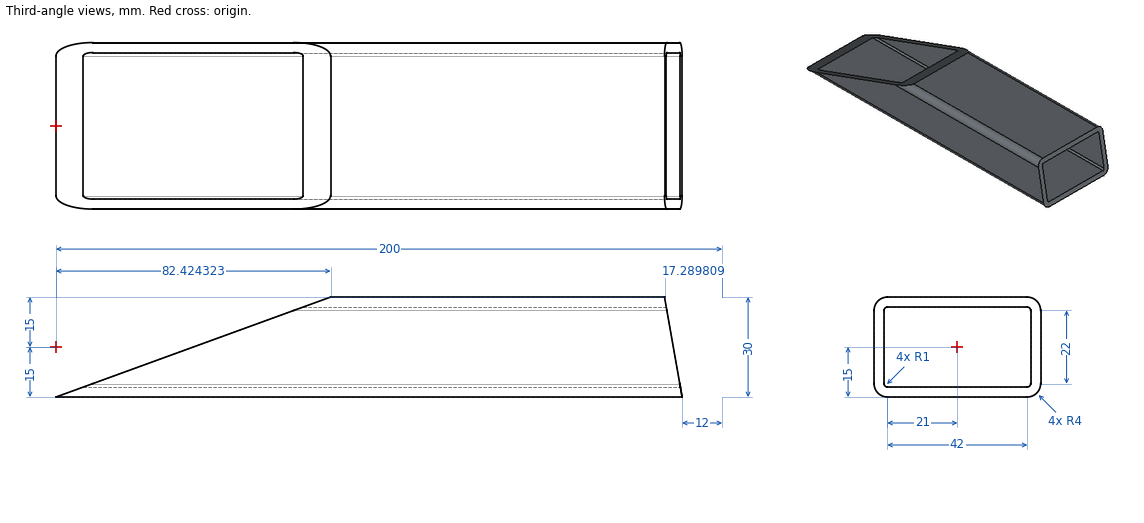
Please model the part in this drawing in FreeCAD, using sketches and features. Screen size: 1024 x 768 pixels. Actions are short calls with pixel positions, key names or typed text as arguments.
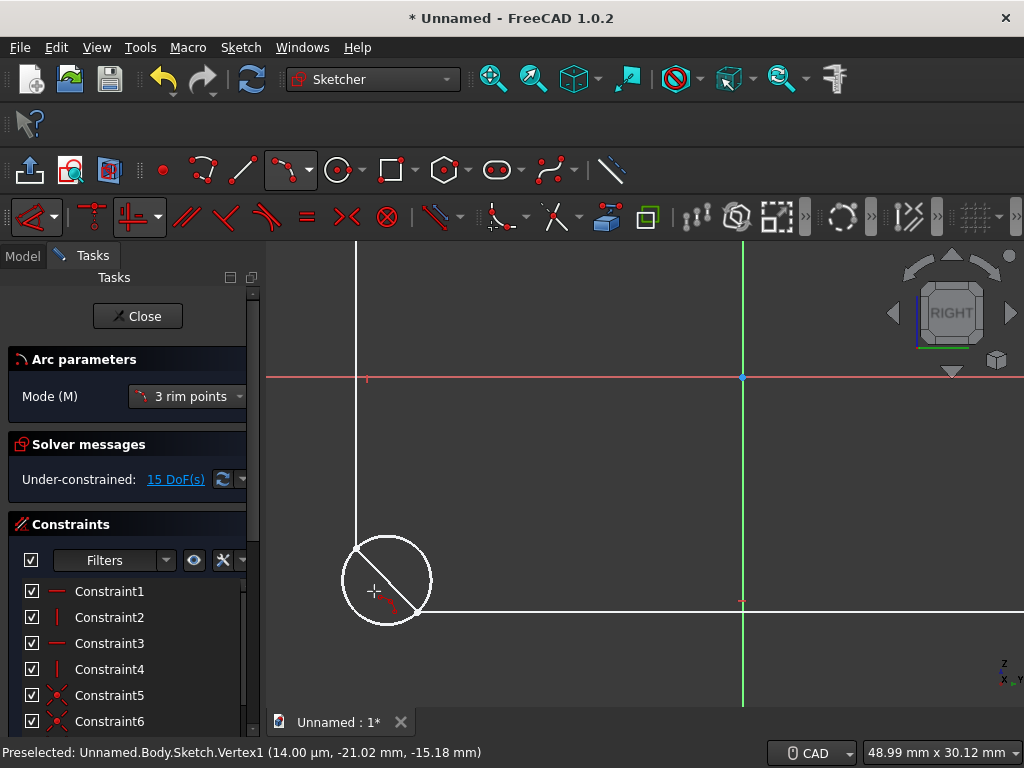
click(374, 591)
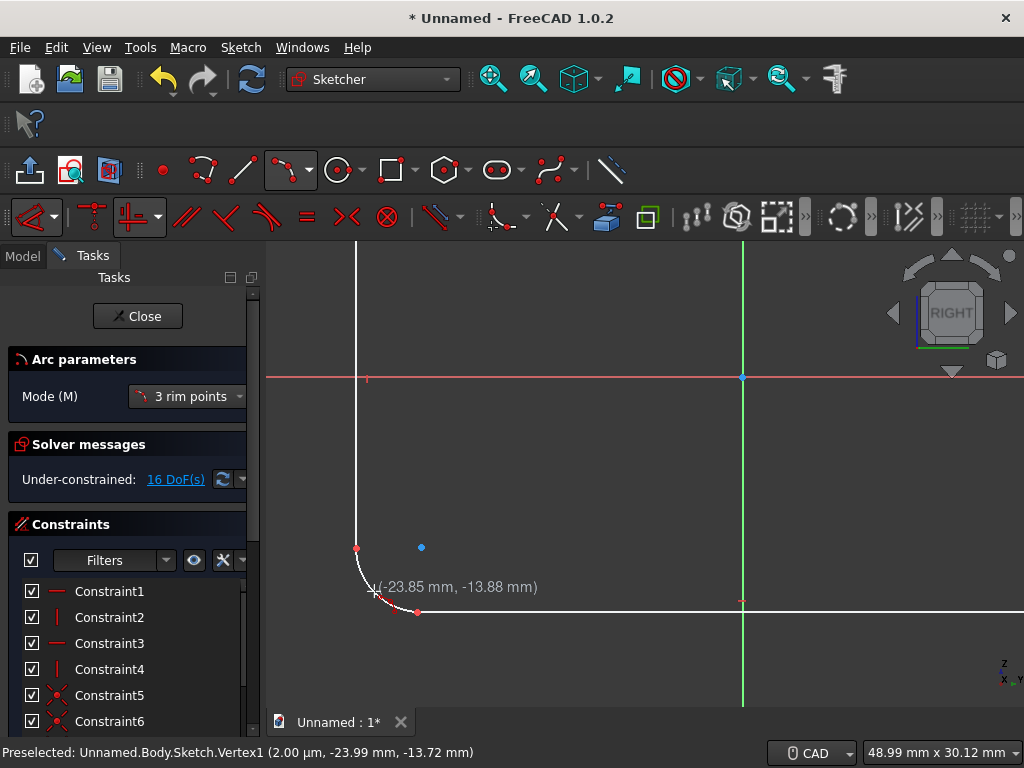
click(244, 170)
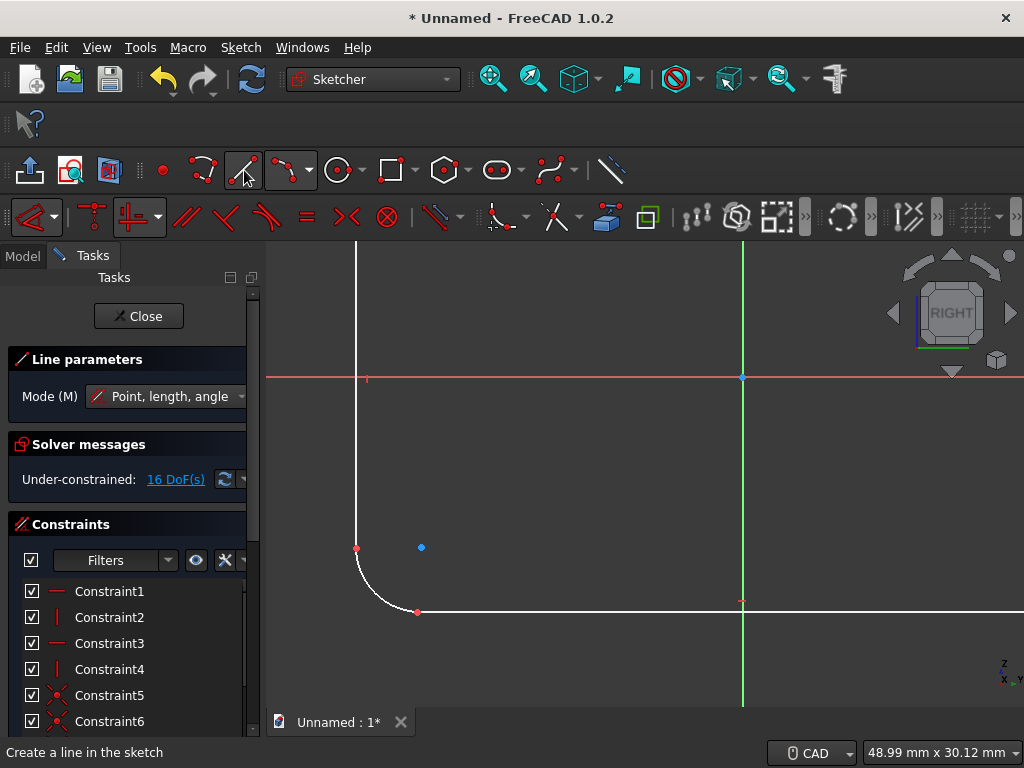
scroll(374, 592, down, 3)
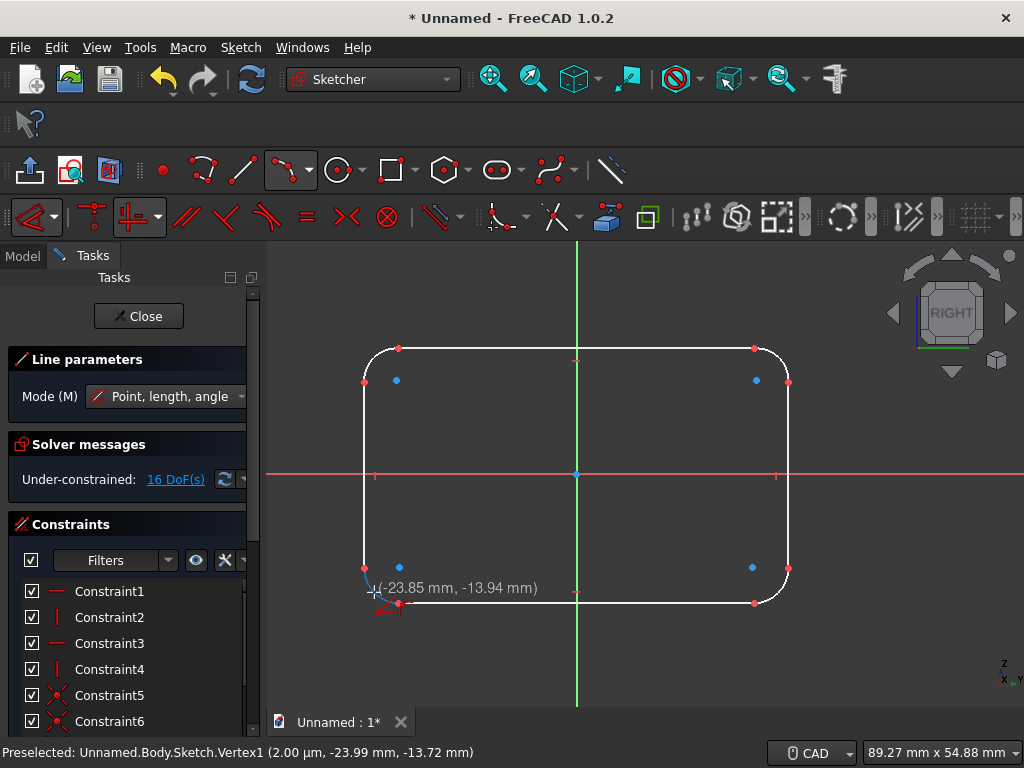
scroll(755, 576, up, 4)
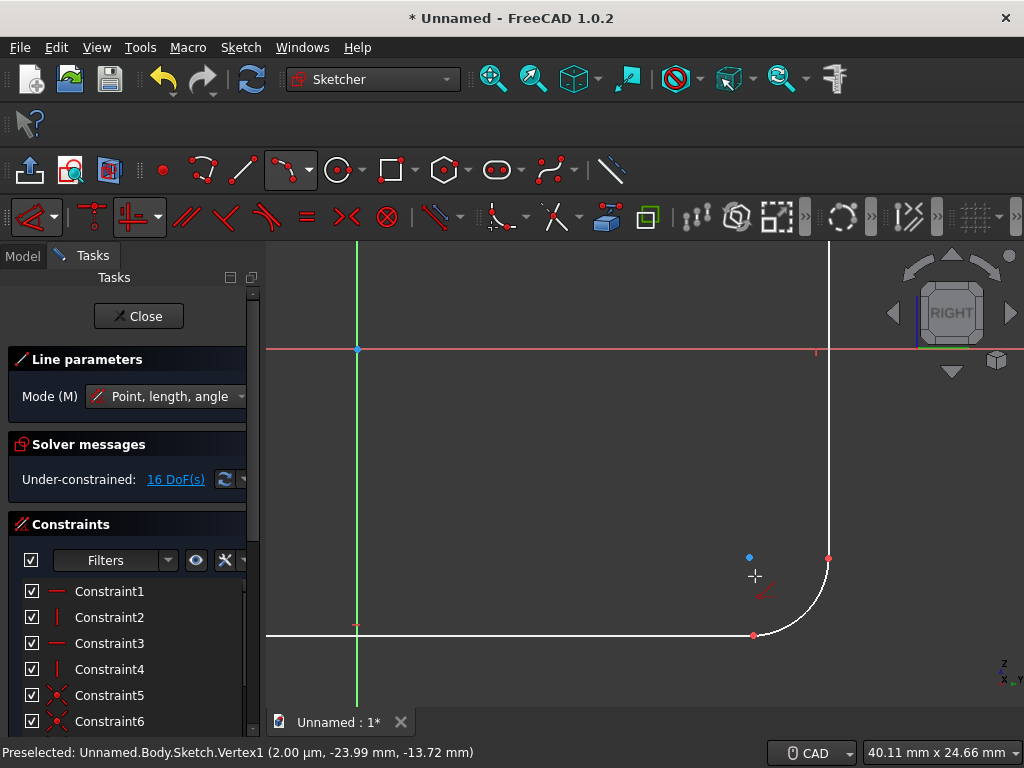
click(754, 576)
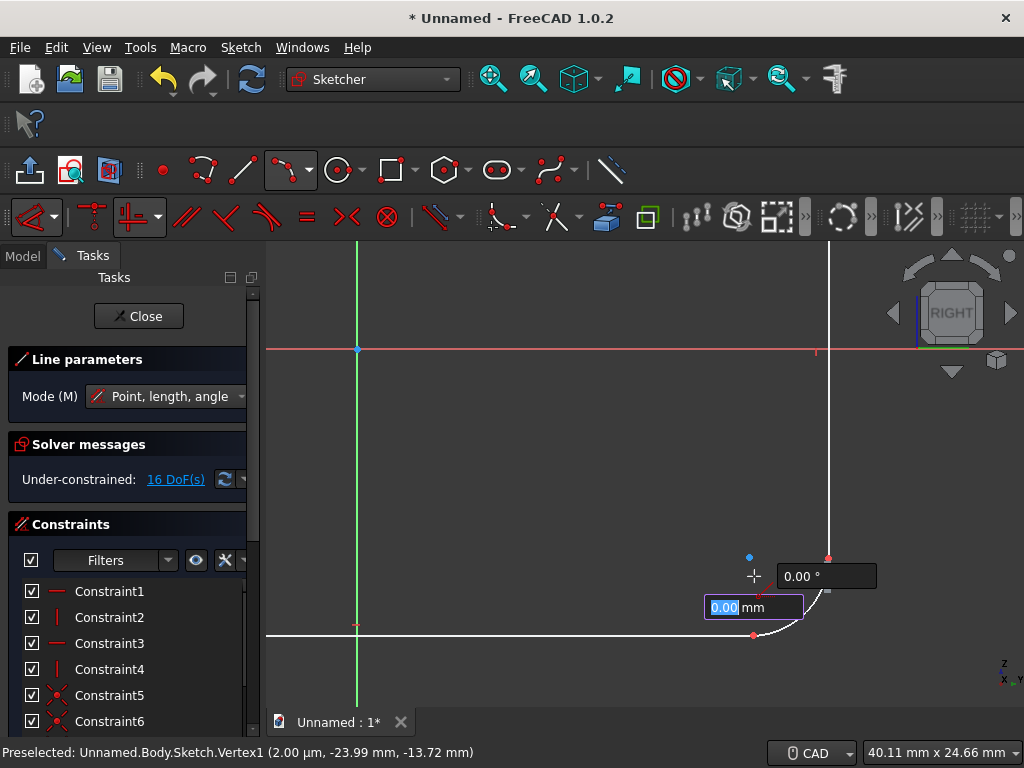
scroll(756, 576, down, 4)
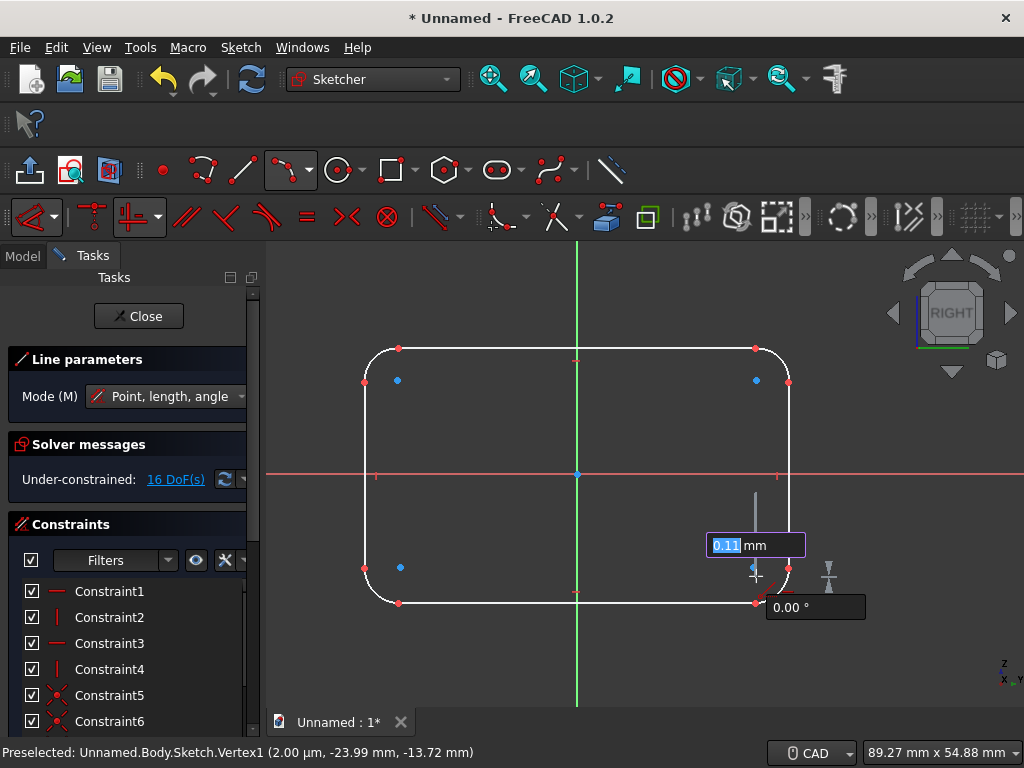
scroll(399, 576, up, 4)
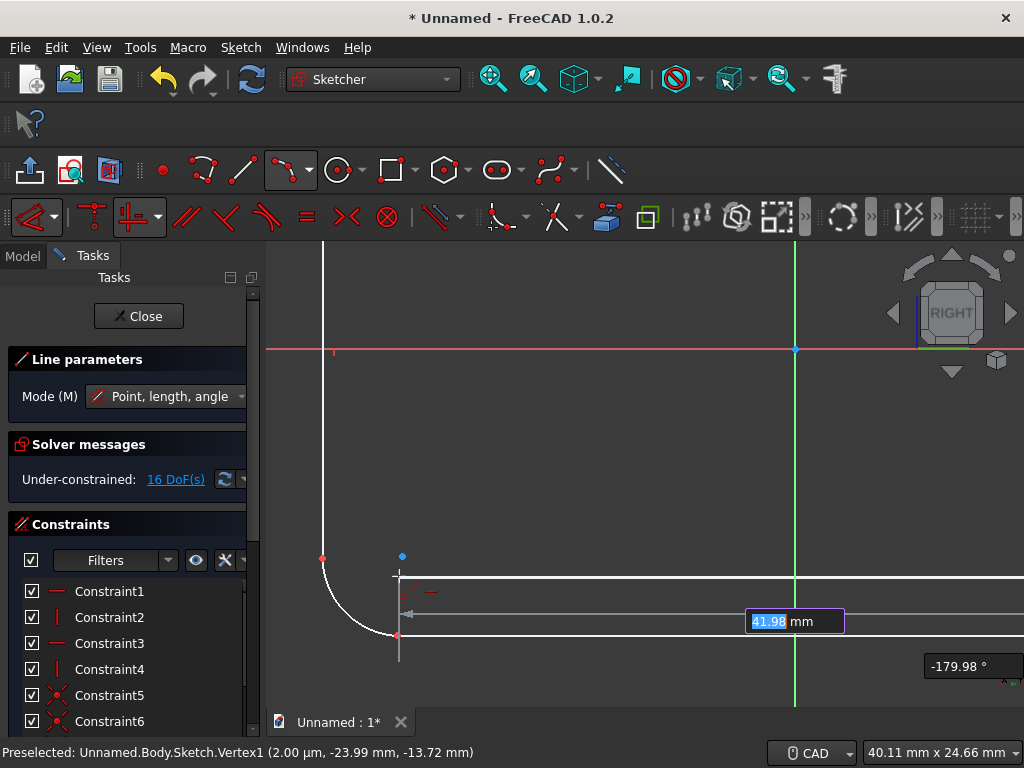
click(398, 576)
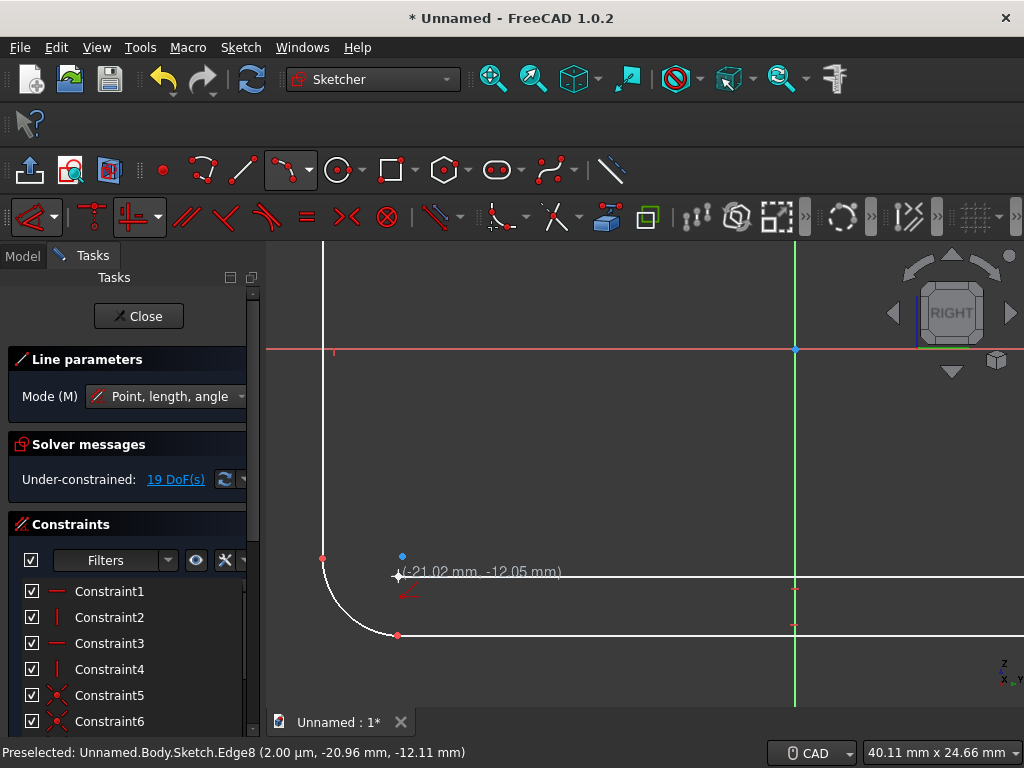
click(379, 557)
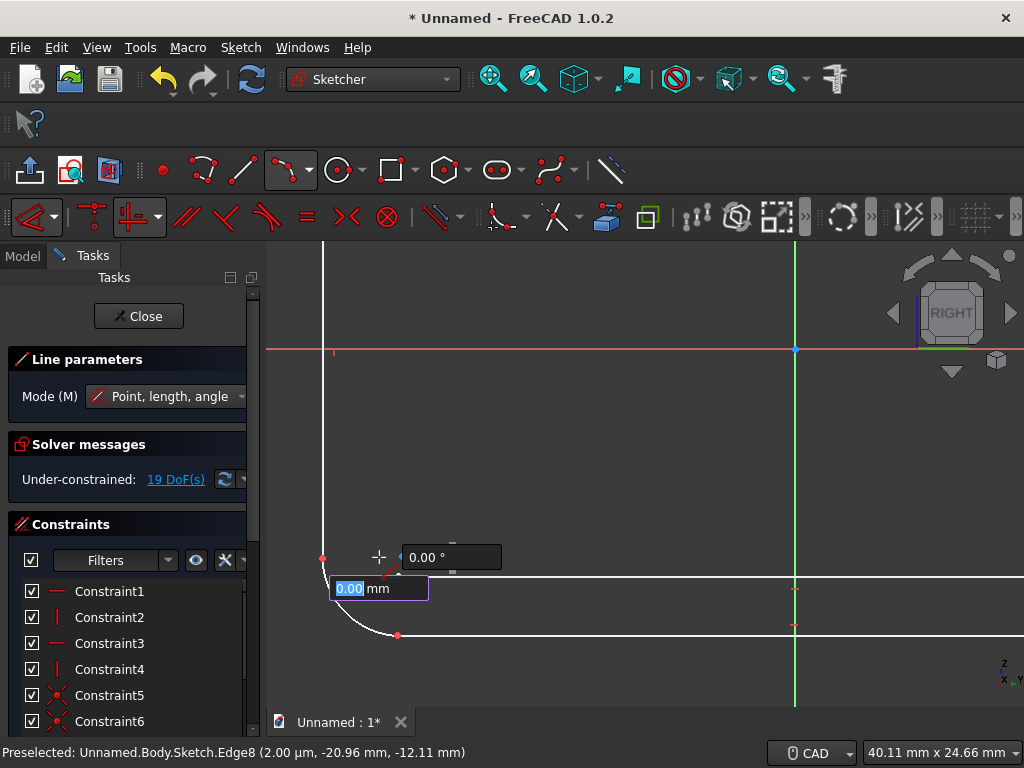
scroll(398, 576, down, 4)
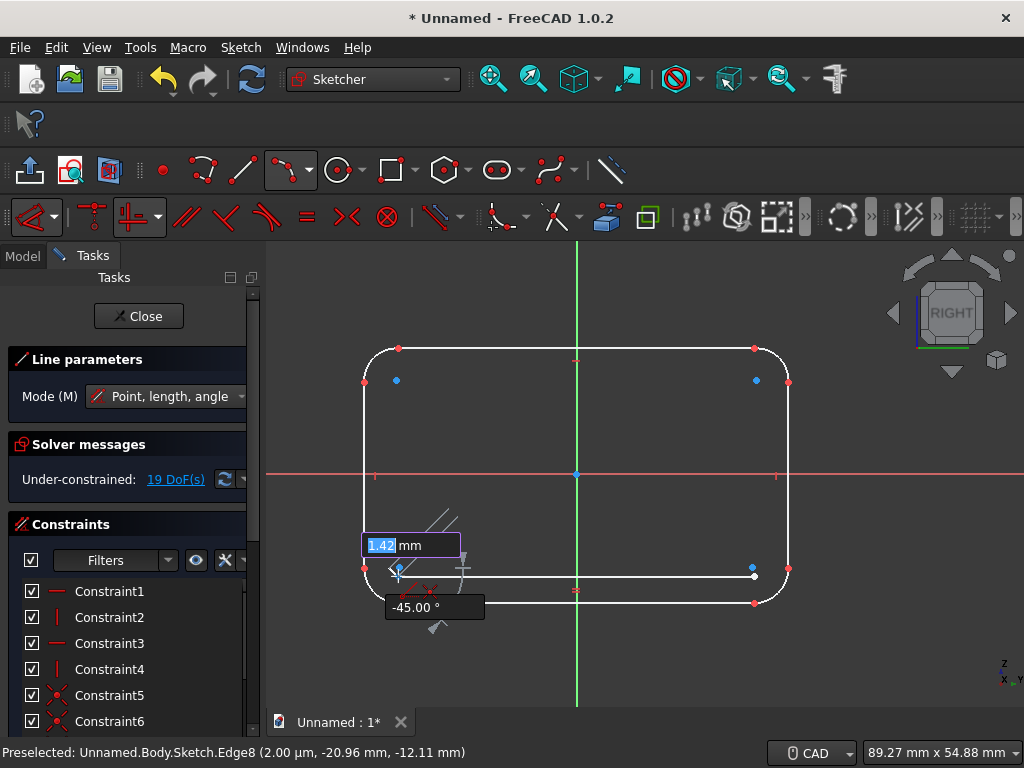
scroll(390, 381, up, 4)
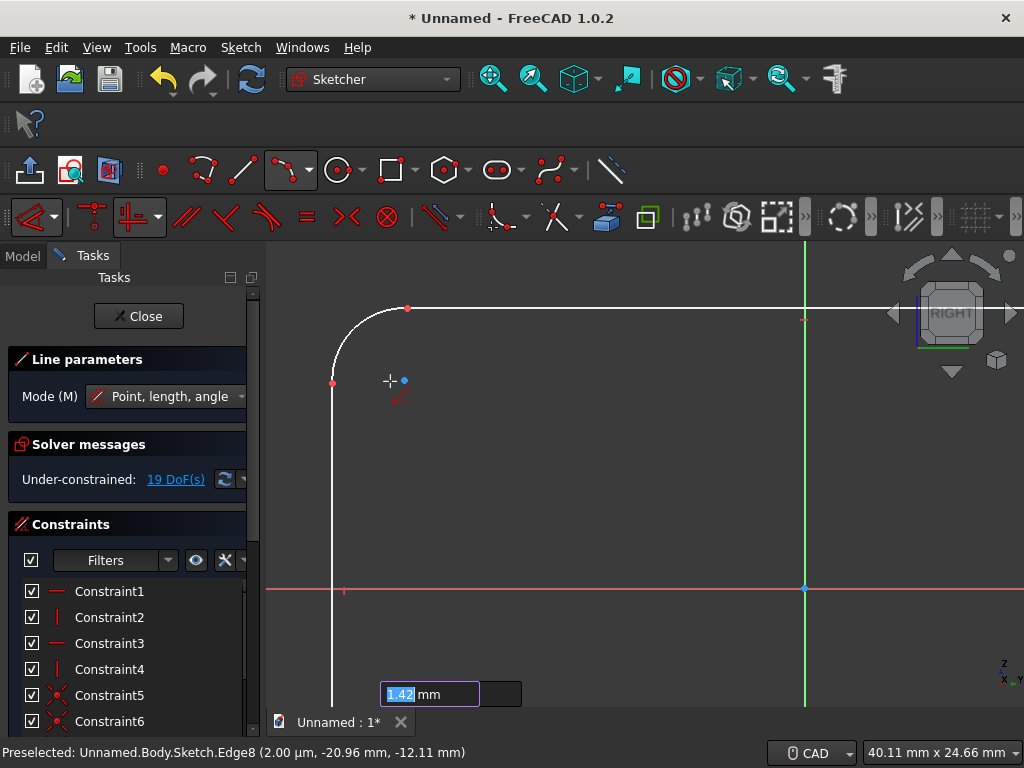
click(389, 381)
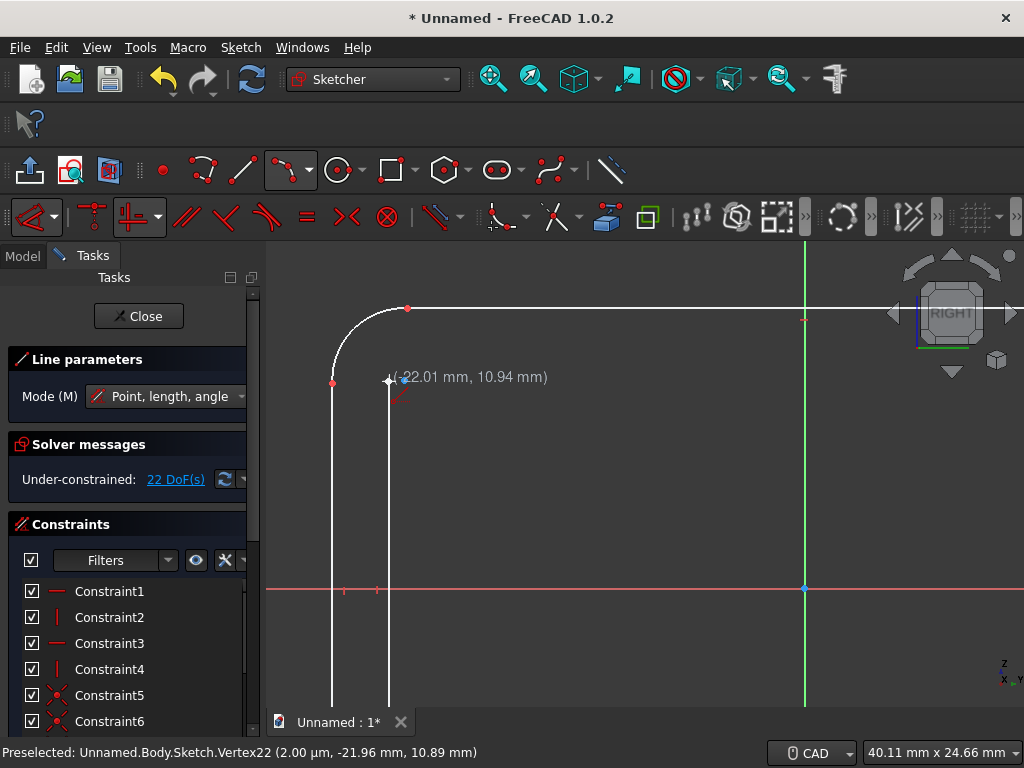
click(408, 362)